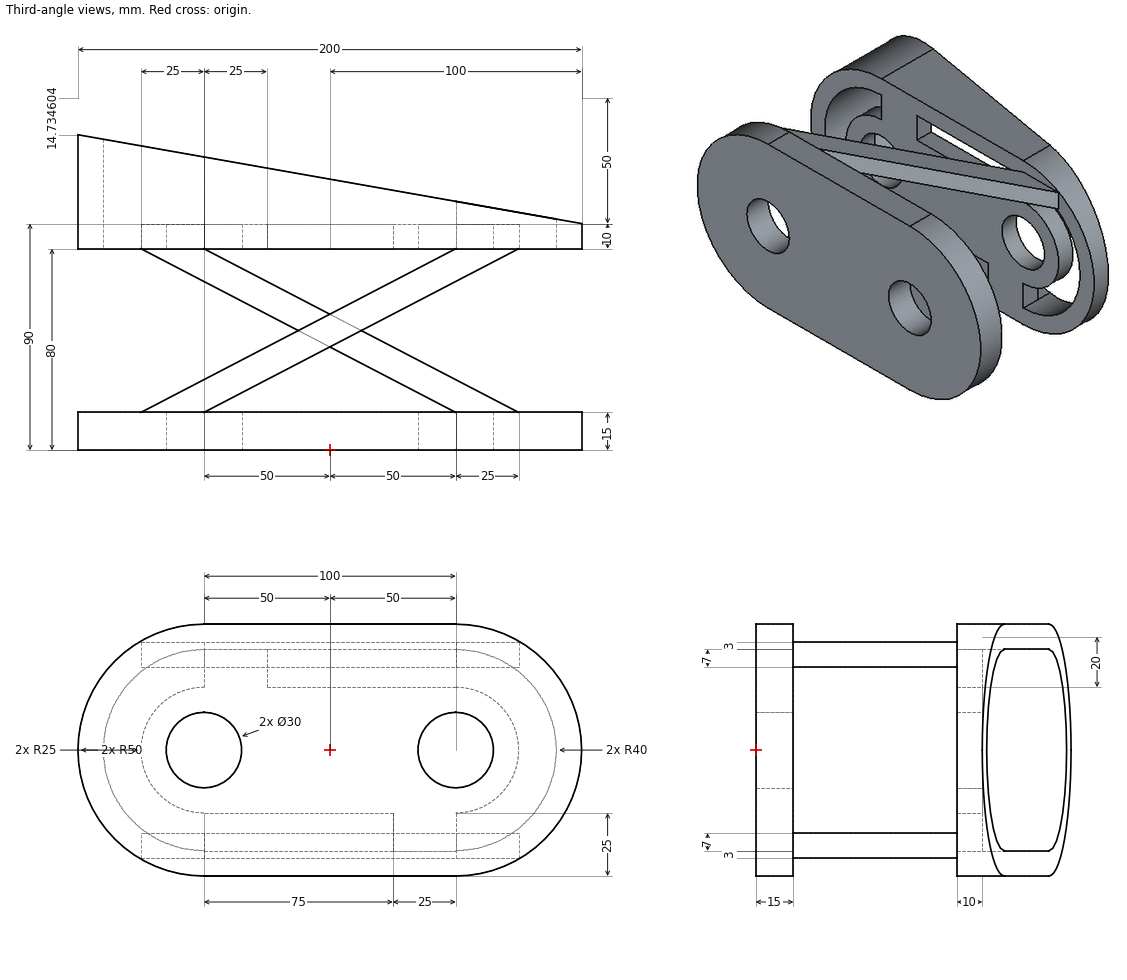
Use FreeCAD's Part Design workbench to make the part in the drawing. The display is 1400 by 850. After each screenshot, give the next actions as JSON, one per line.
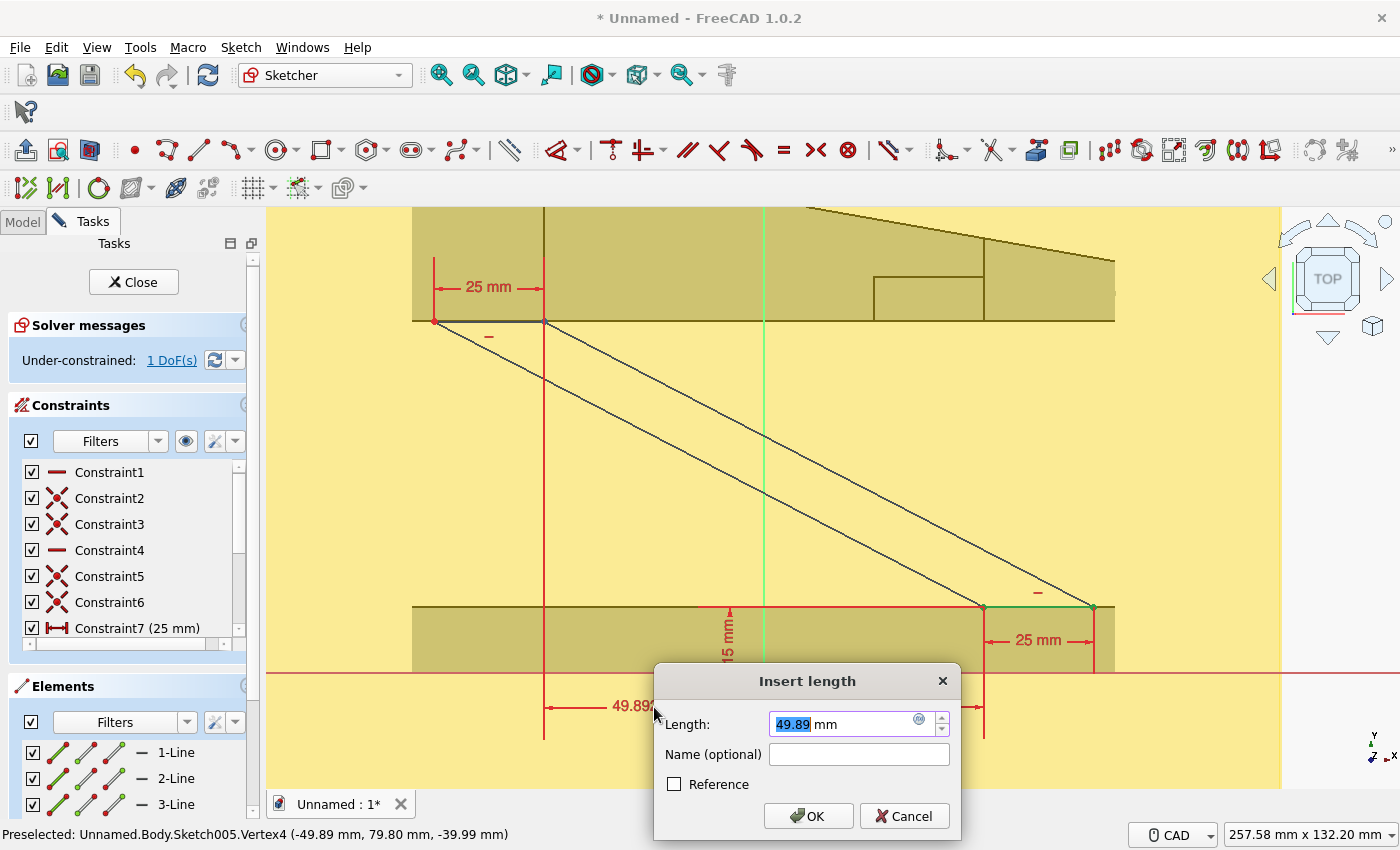
{"action": "type", "text": "50"}
{"action": "key", "text": "Return"}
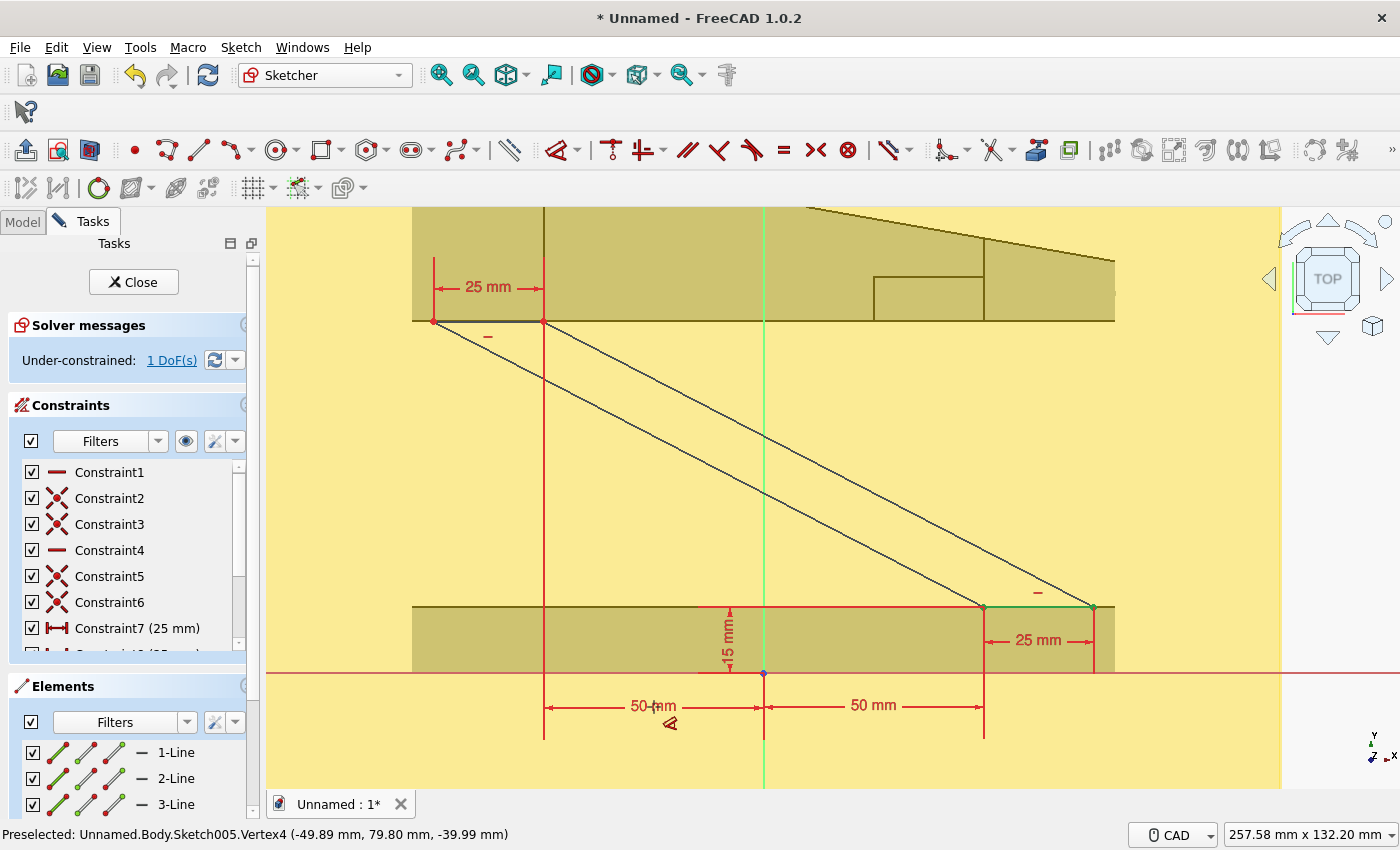
{"action": "left_click", "coordinate": [544, 322]}
{"action": "left_click", "coordinate": [510, 498]}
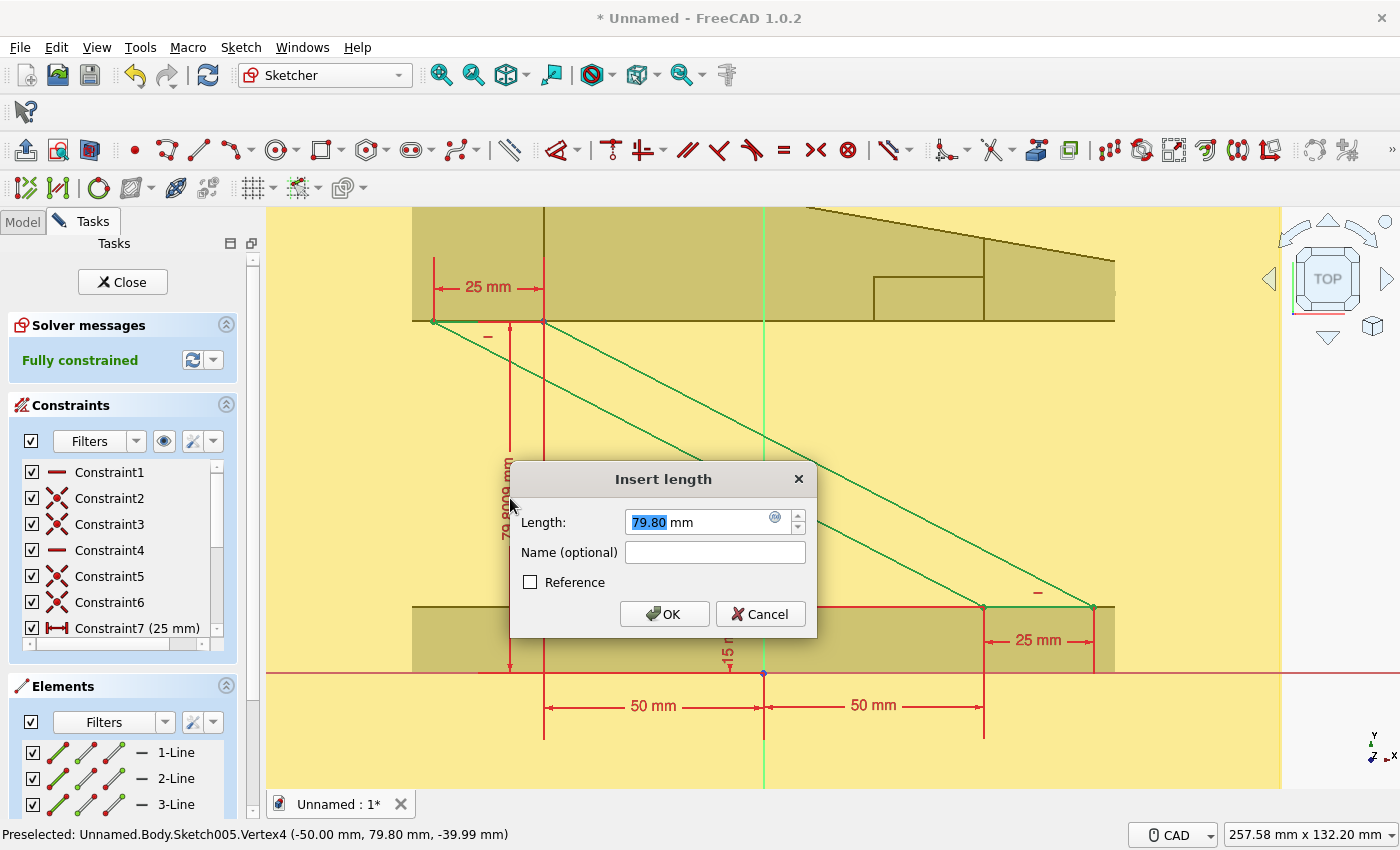
{"action": "type", "text": "80"}
{"action": "key", "text": "Return"}
{"action": "key", "text": "Escape"}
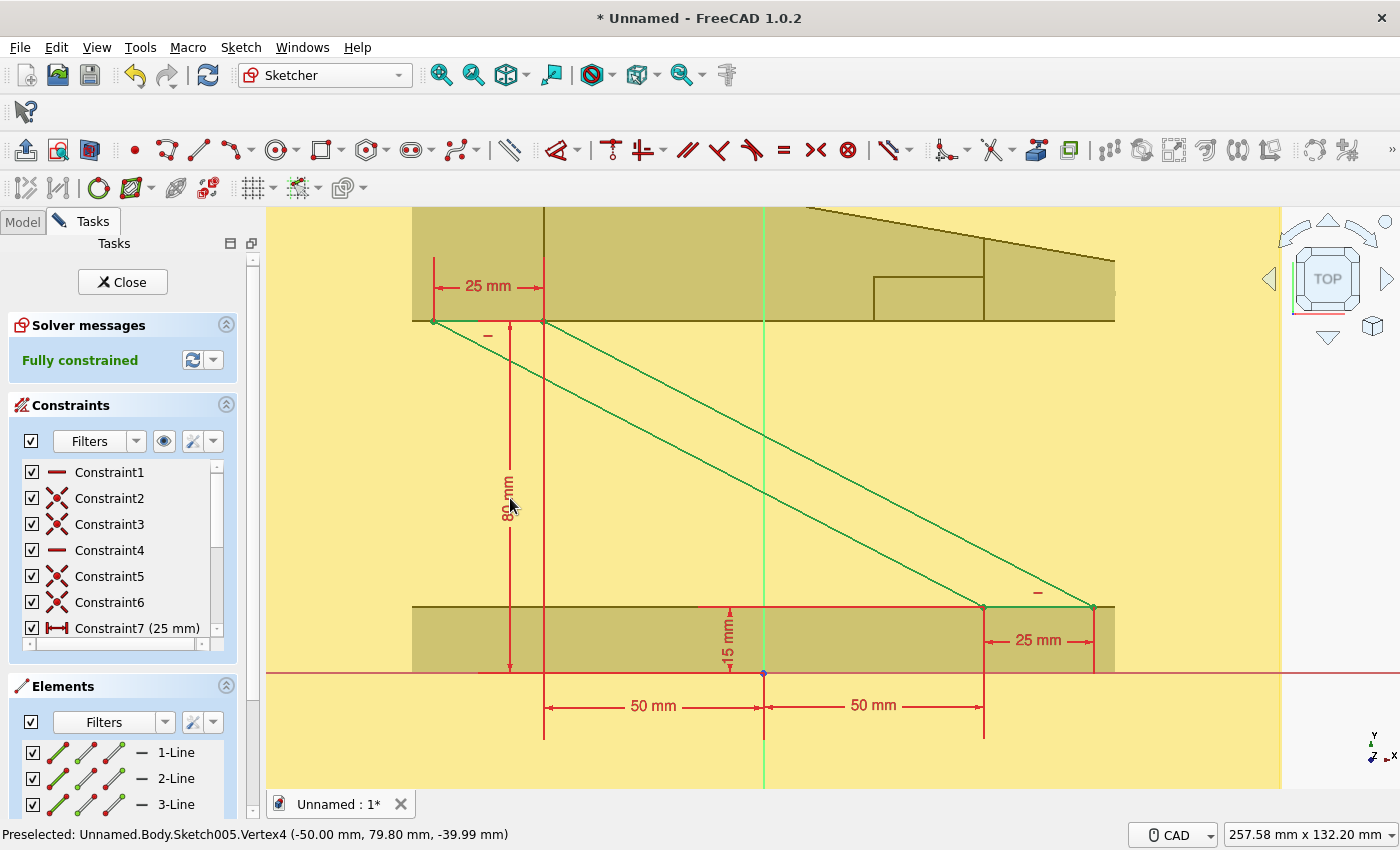
{"action": "left_click", "coordinate": [123, 282]}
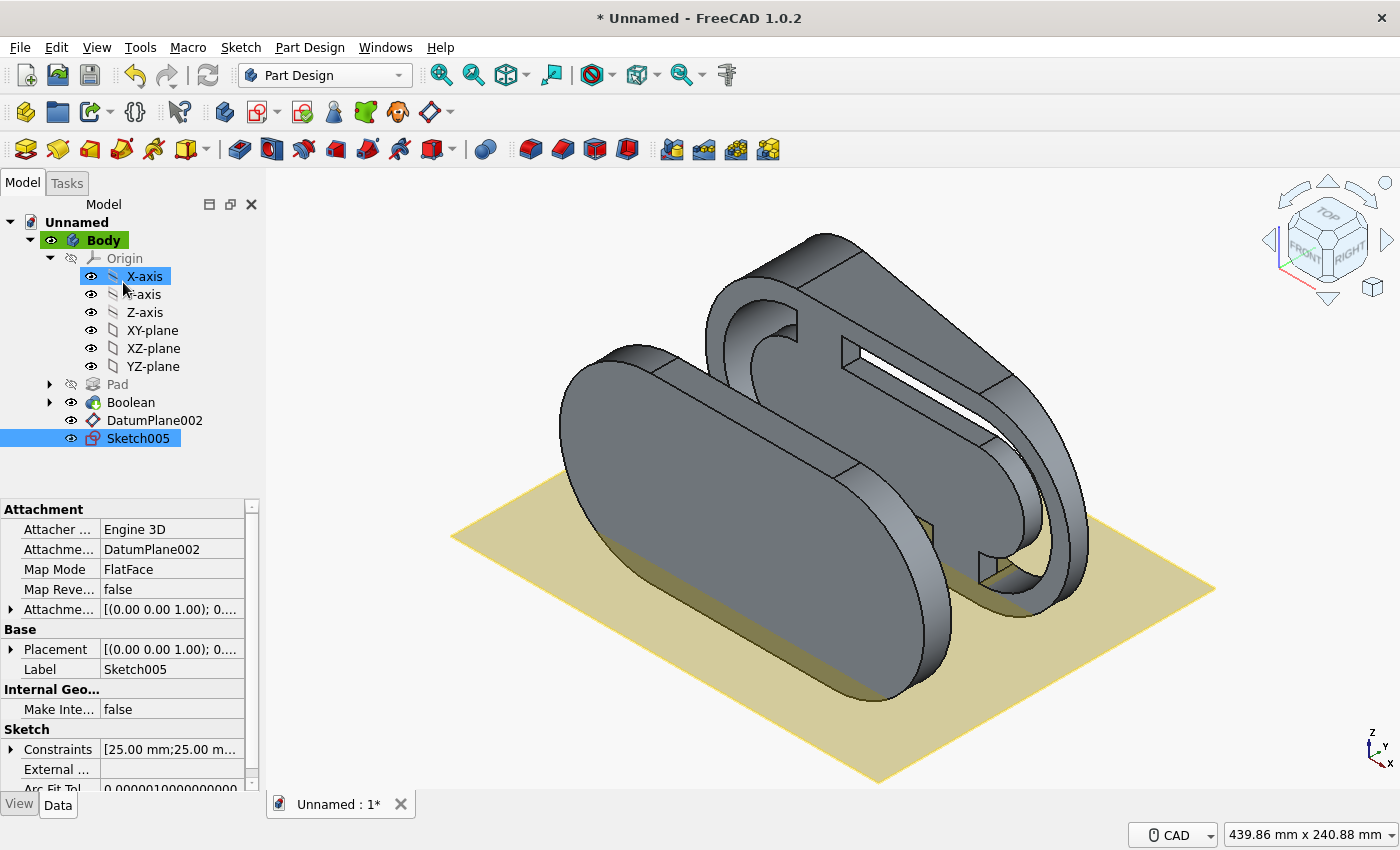
{"action": "left_click", "coordinate": [26, 150]}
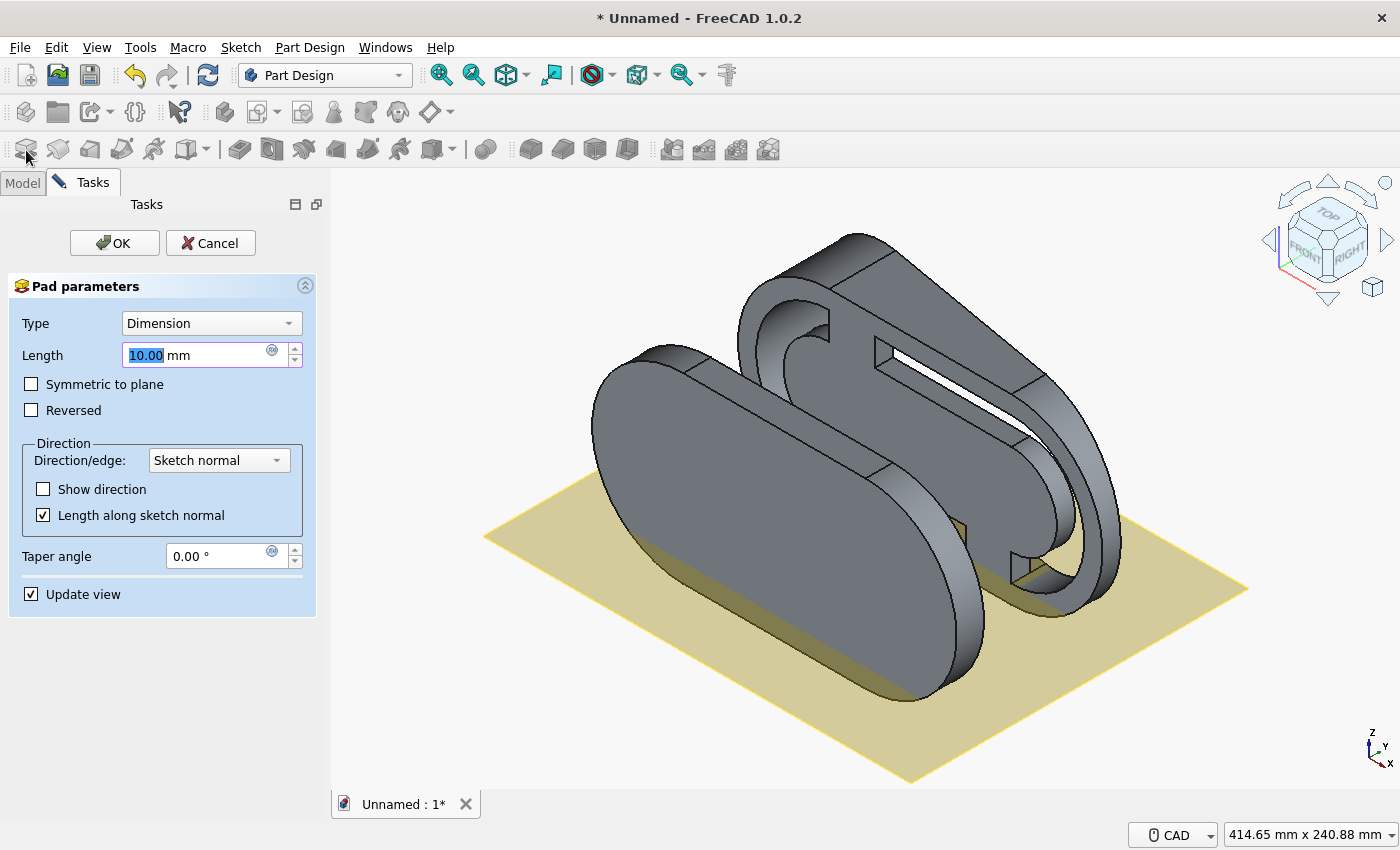
{"action": "left_click", "coordinate": [212, 324]}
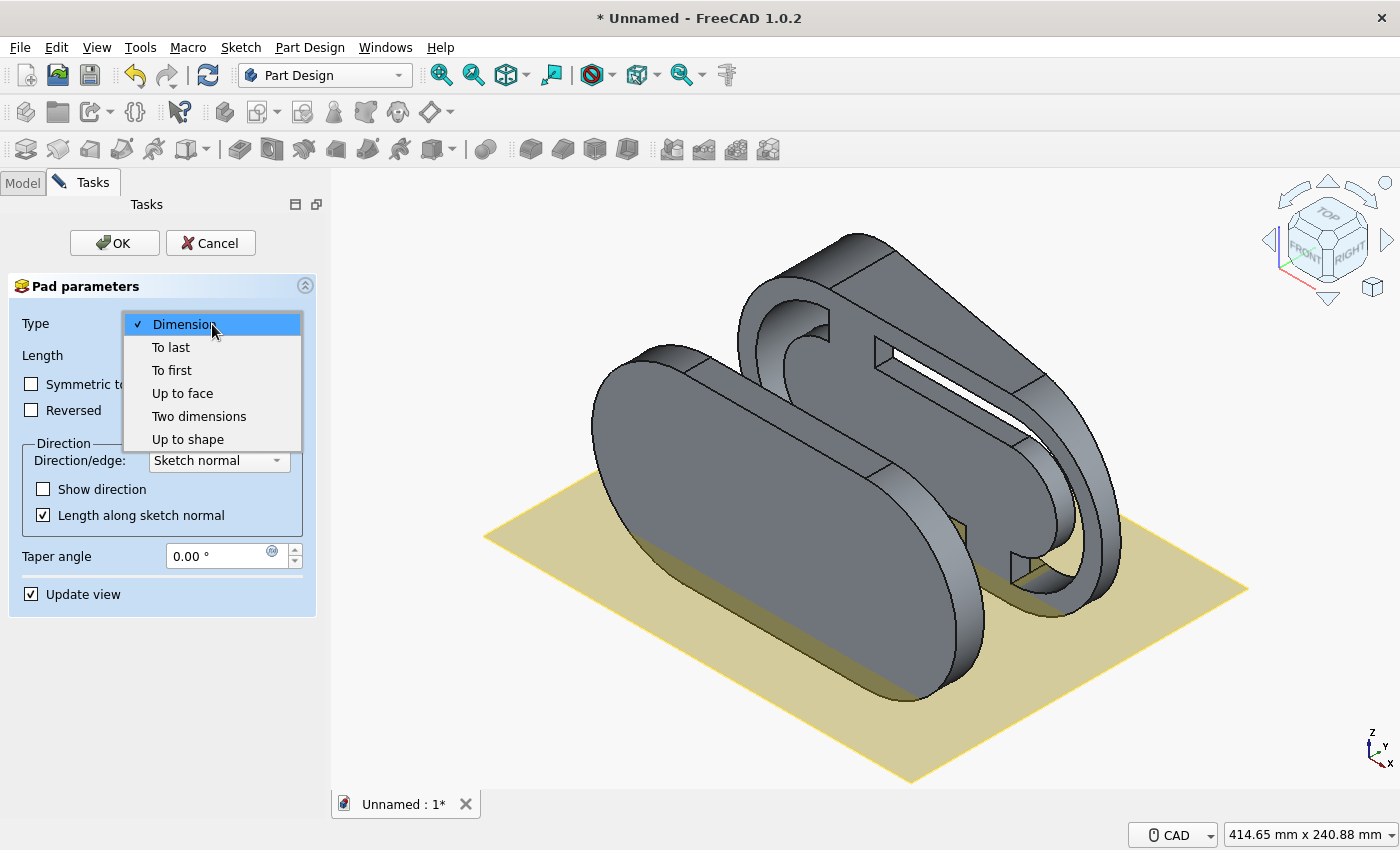
{"action": "left_click", "coordinate": [212, 416]}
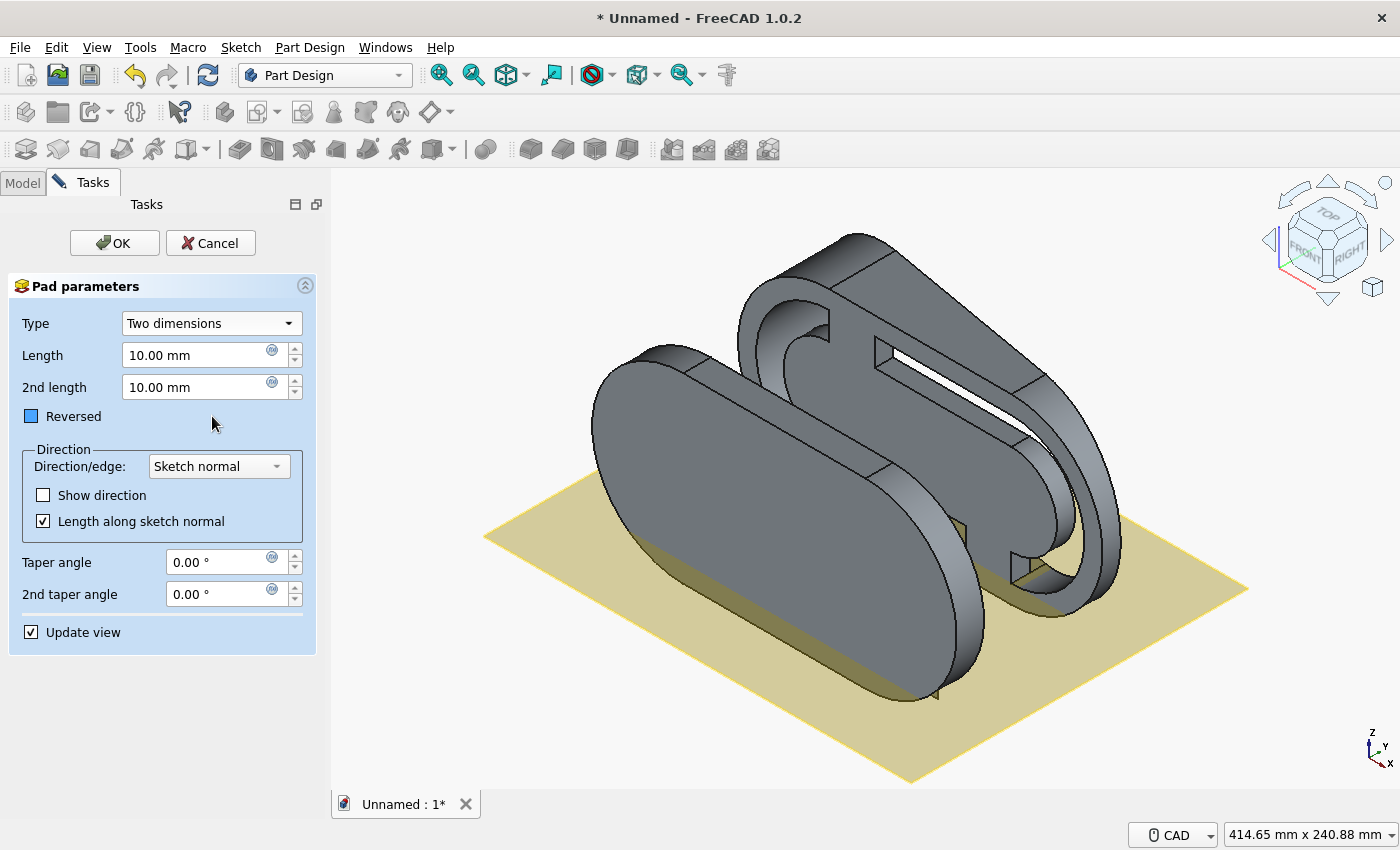
{"action": "triple_click", "coordinate": [204, 355]}